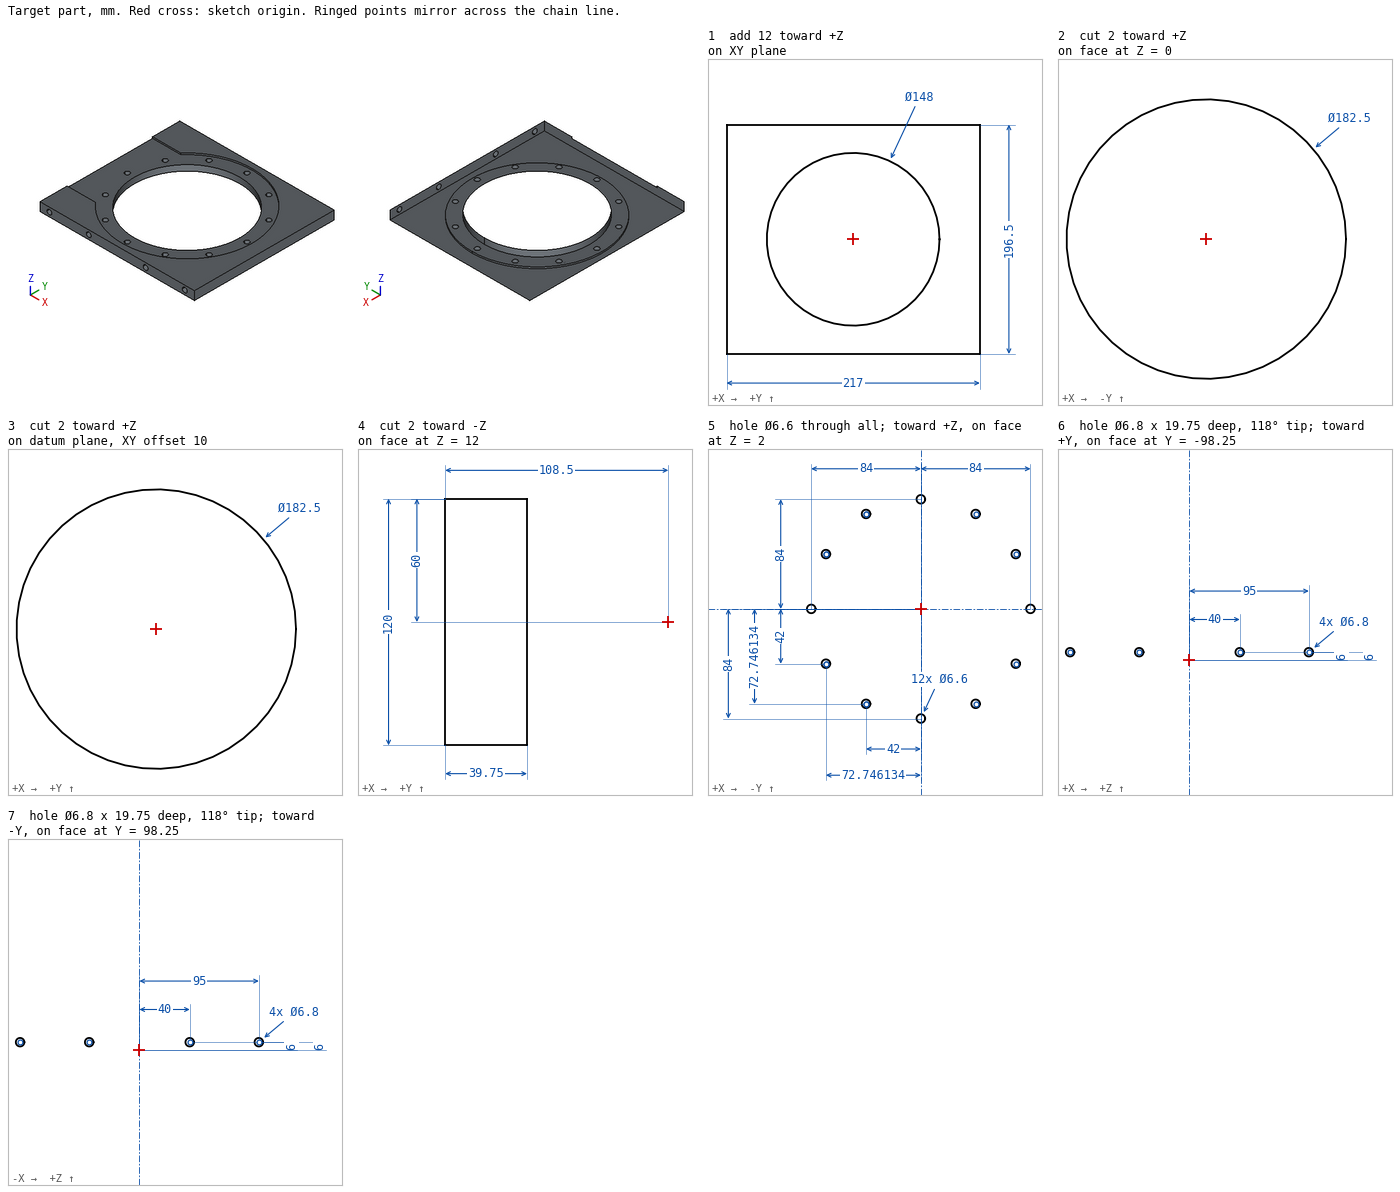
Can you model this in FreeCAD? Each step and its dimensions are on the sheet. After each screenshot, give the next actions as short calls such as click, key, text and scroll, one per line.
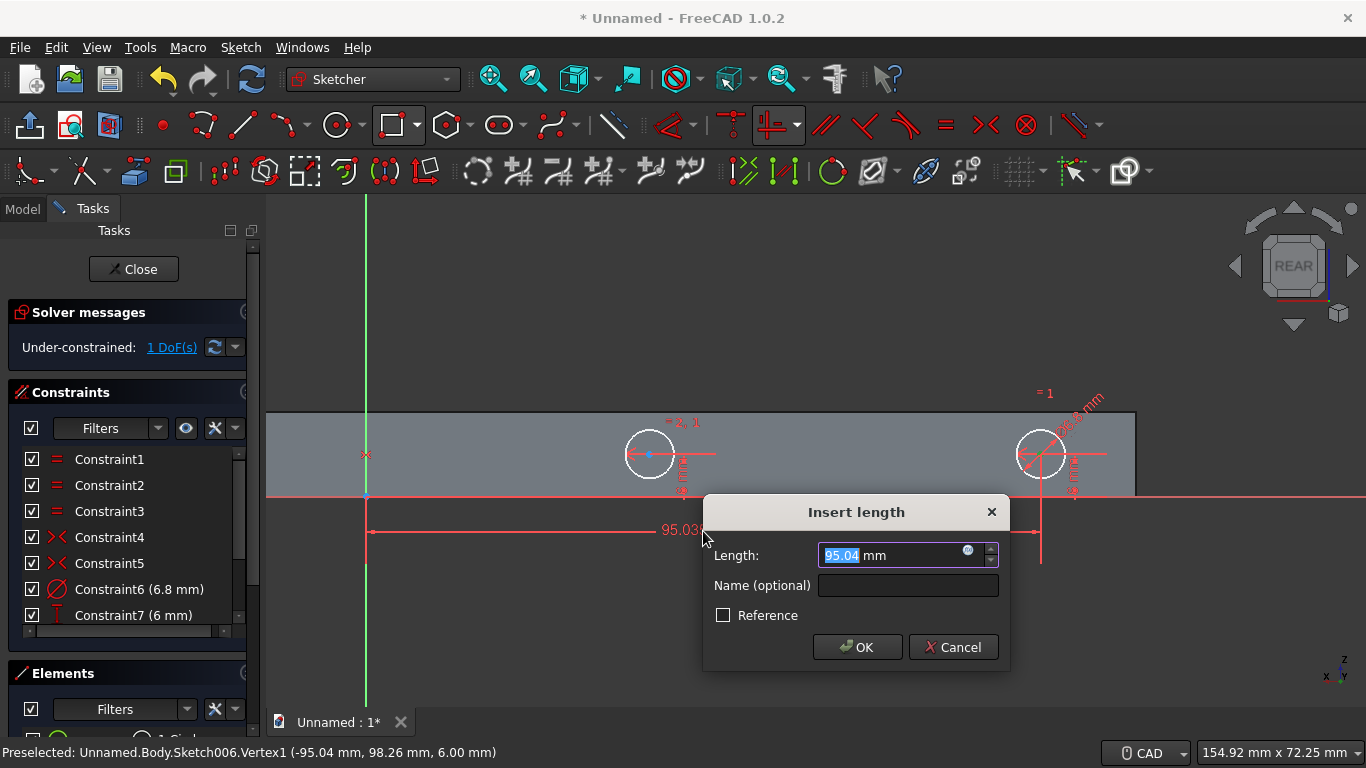
text(95)
key(Return)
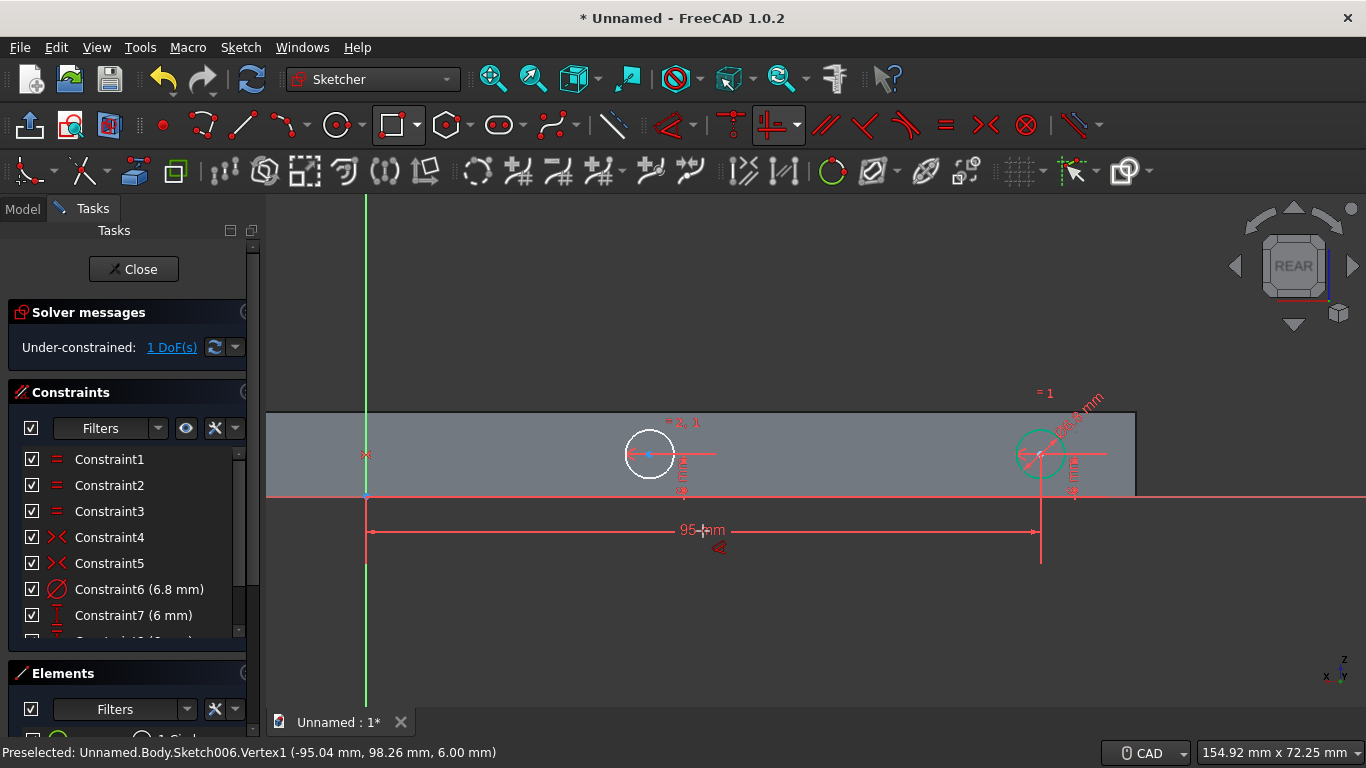
click(650, 454)
click(508, 531)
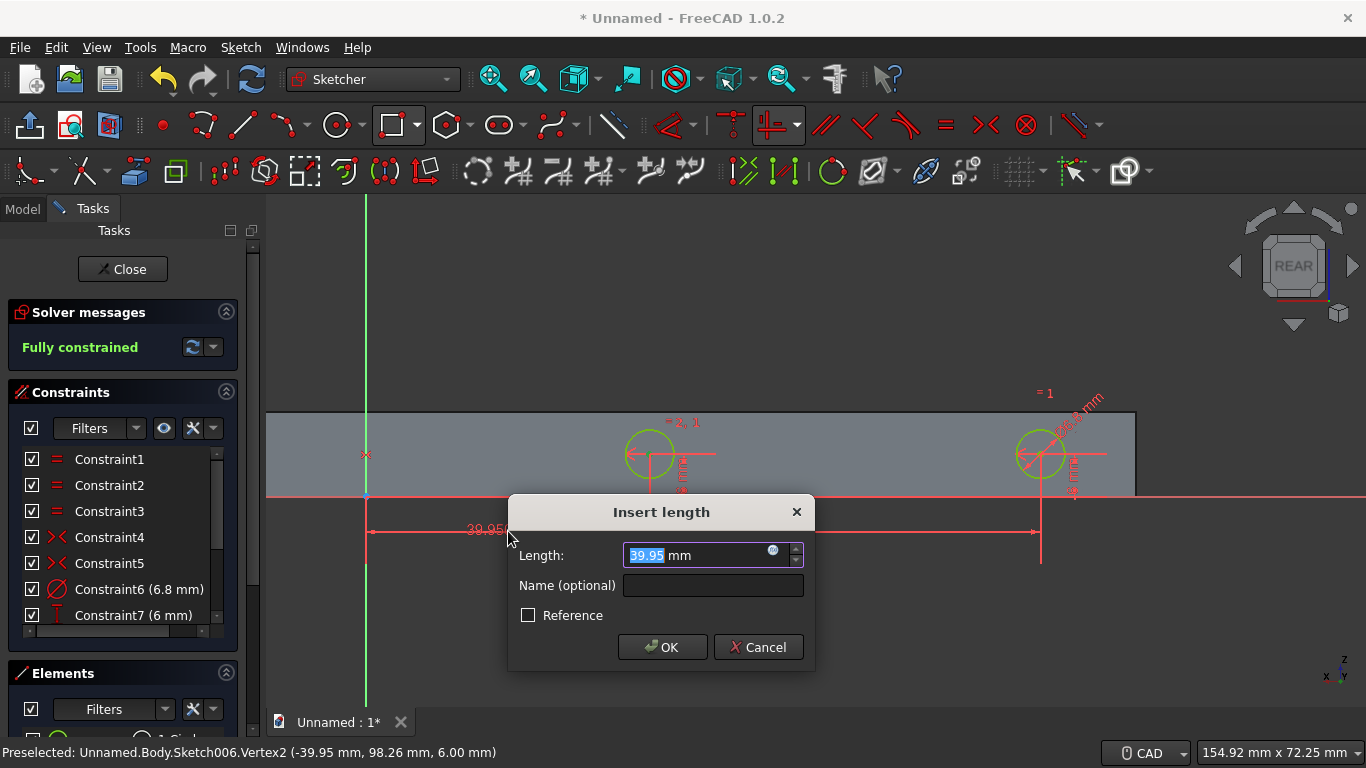
text(40)
key(Return)
key(Escape)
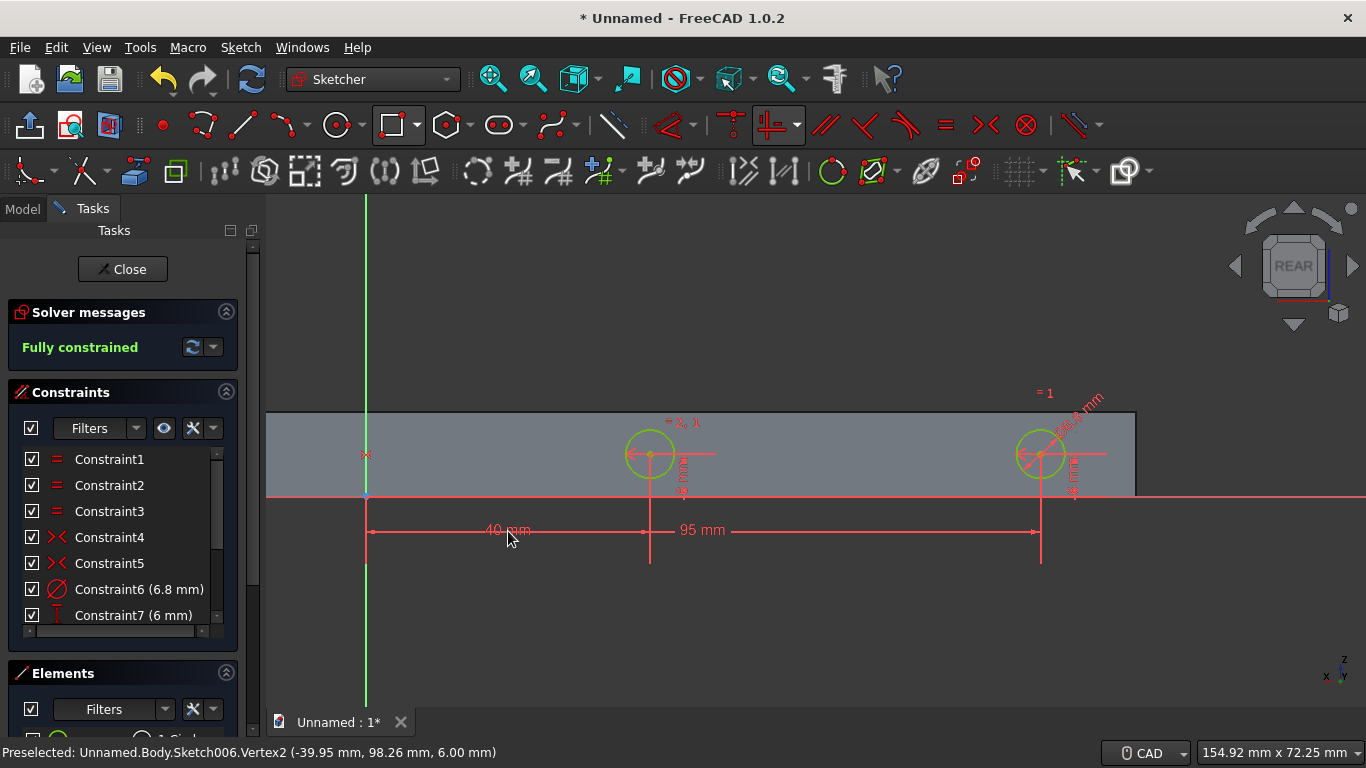
click(123, 269)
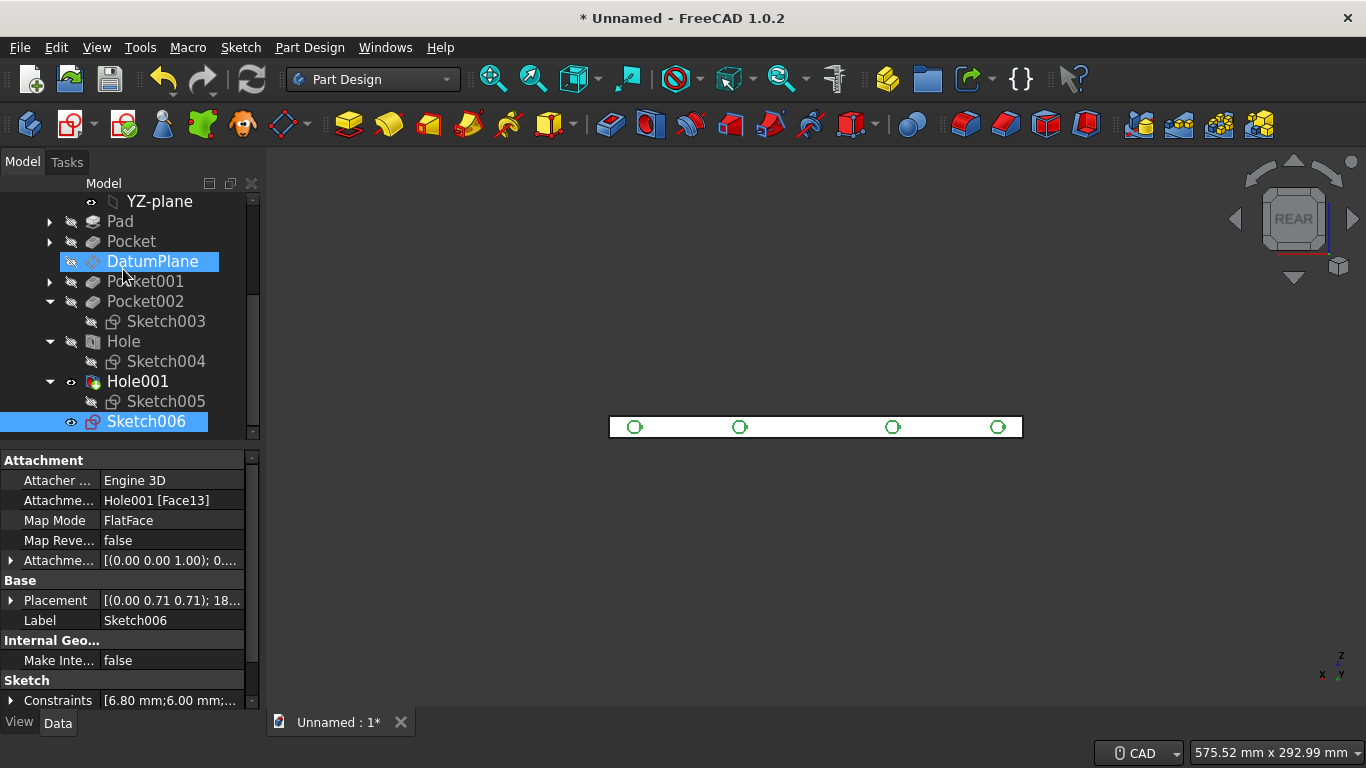
click(652, 124)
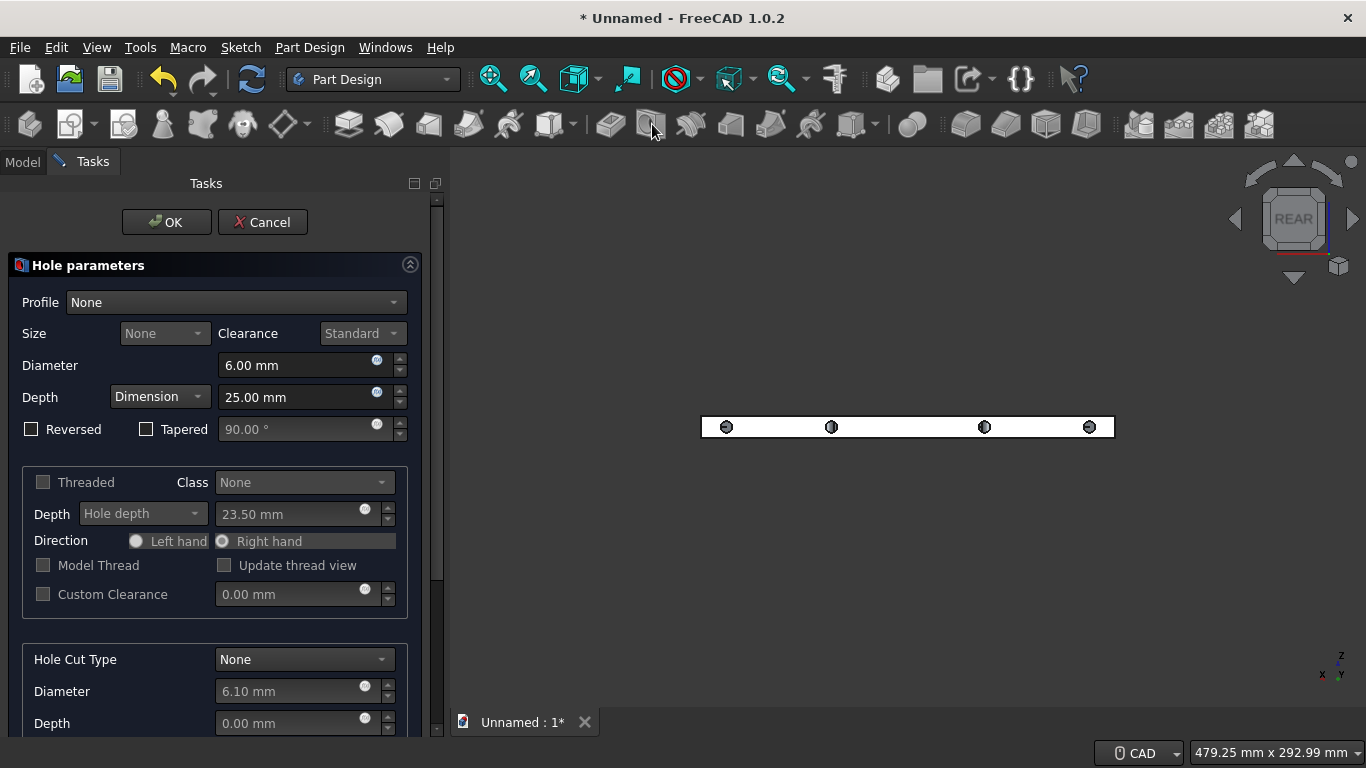
triple_click(305, 365)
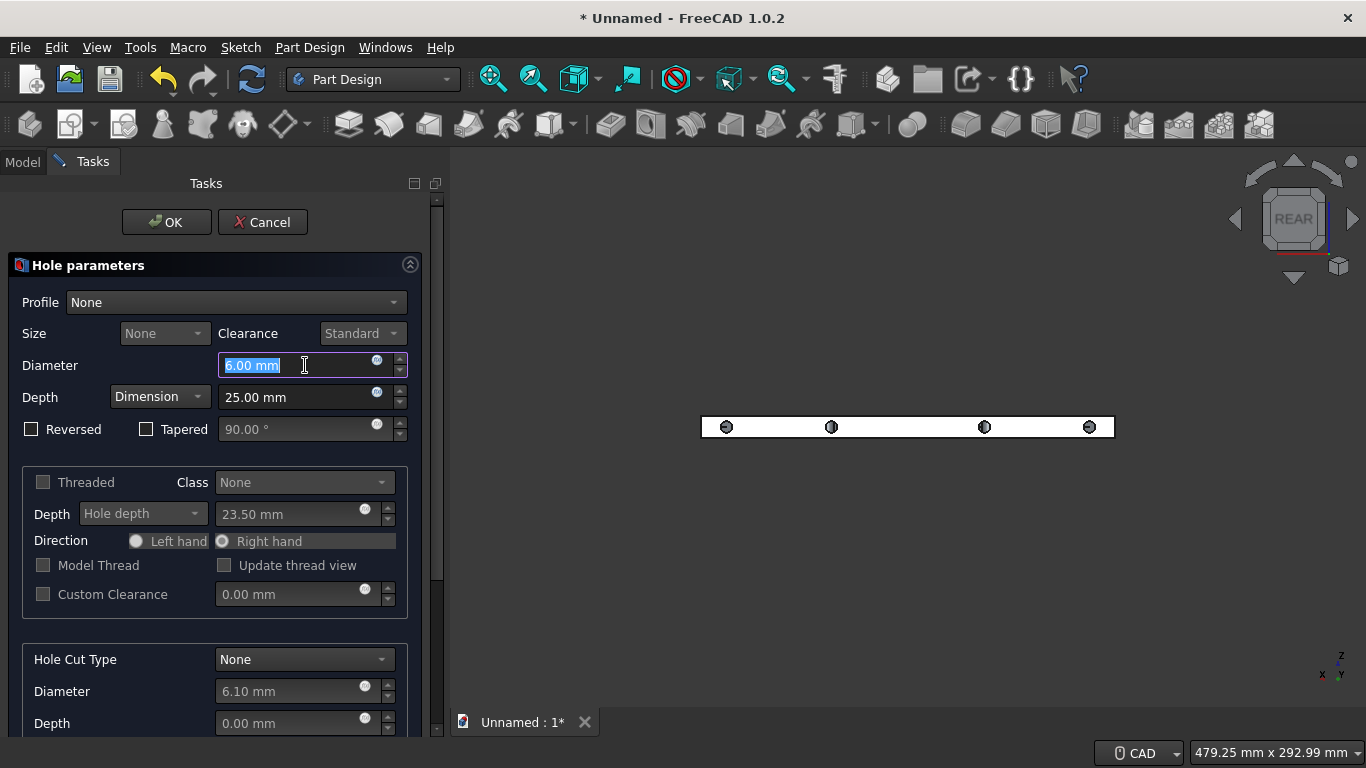
text(6.8)
key(Tab)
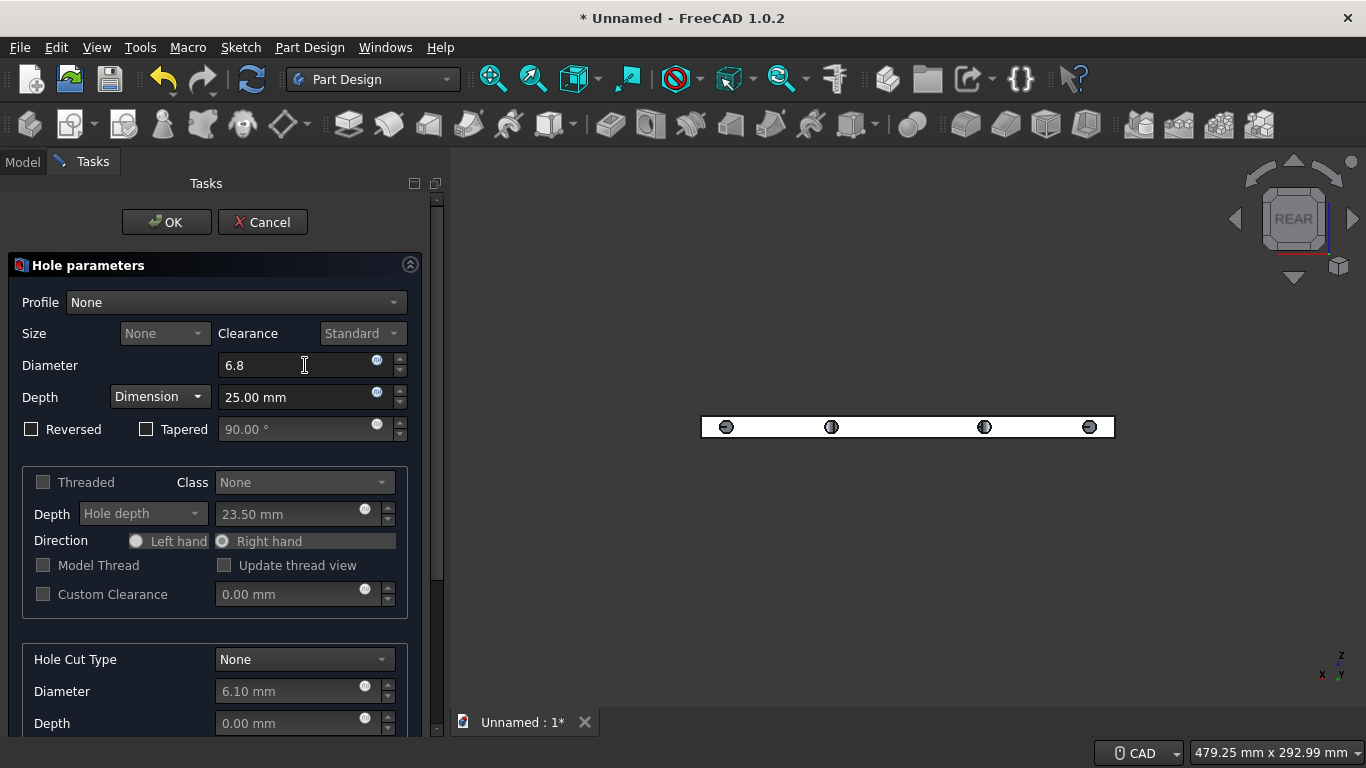
triple_click(305, 397)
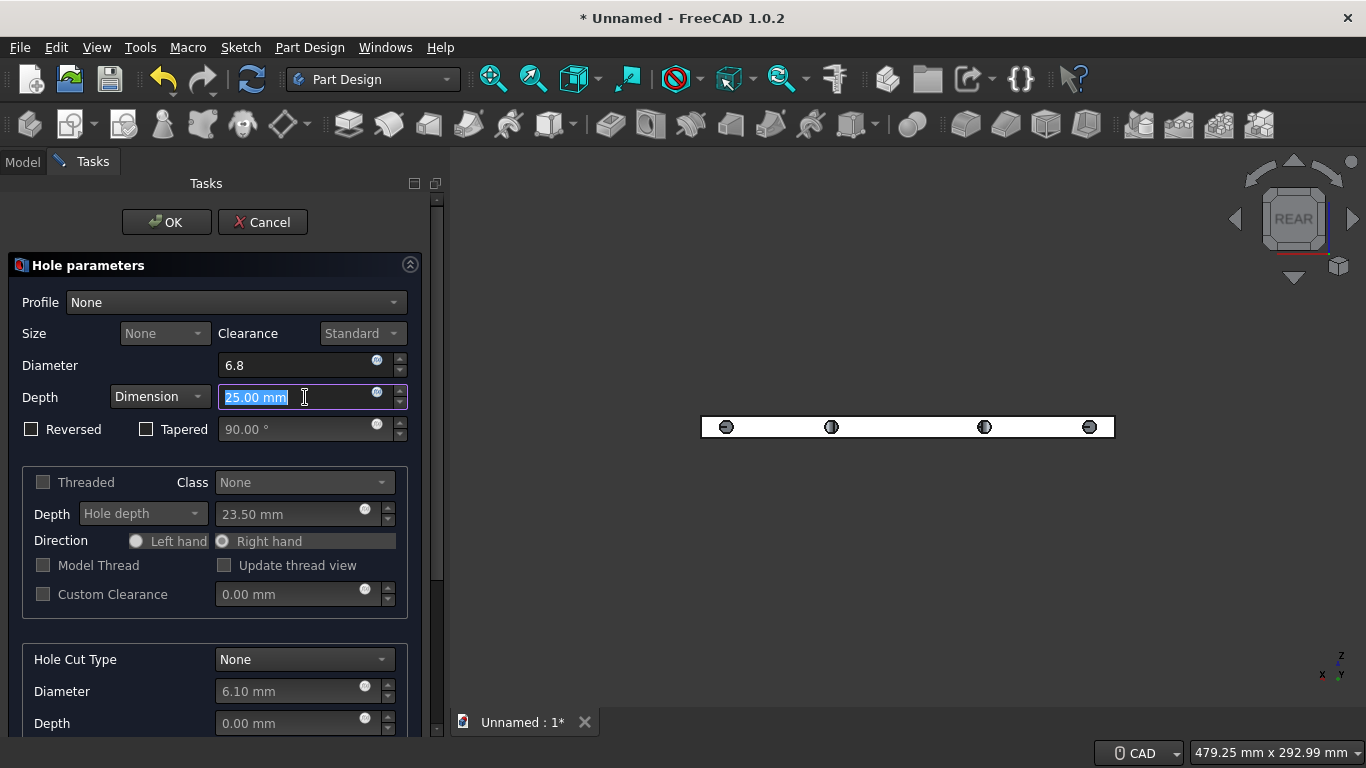
text(19.75)
key(Tab)